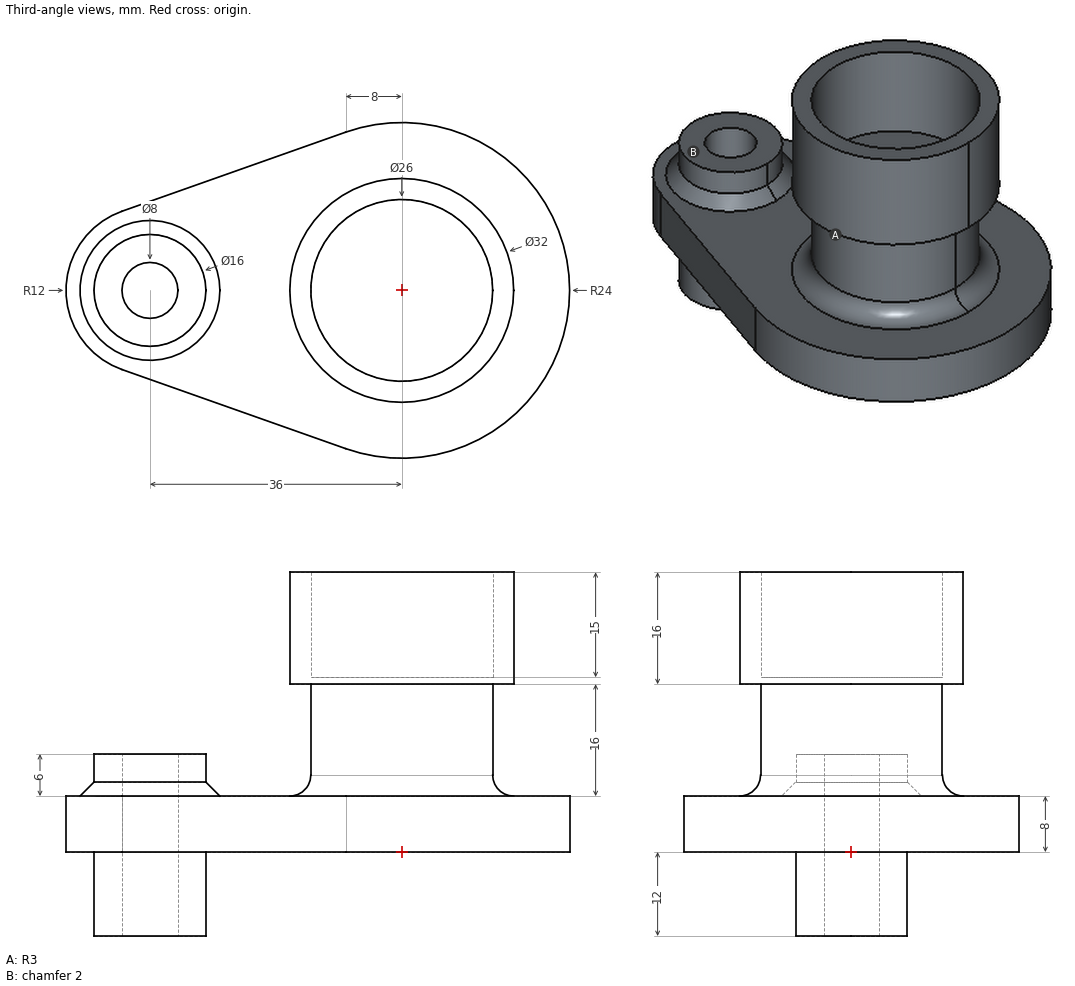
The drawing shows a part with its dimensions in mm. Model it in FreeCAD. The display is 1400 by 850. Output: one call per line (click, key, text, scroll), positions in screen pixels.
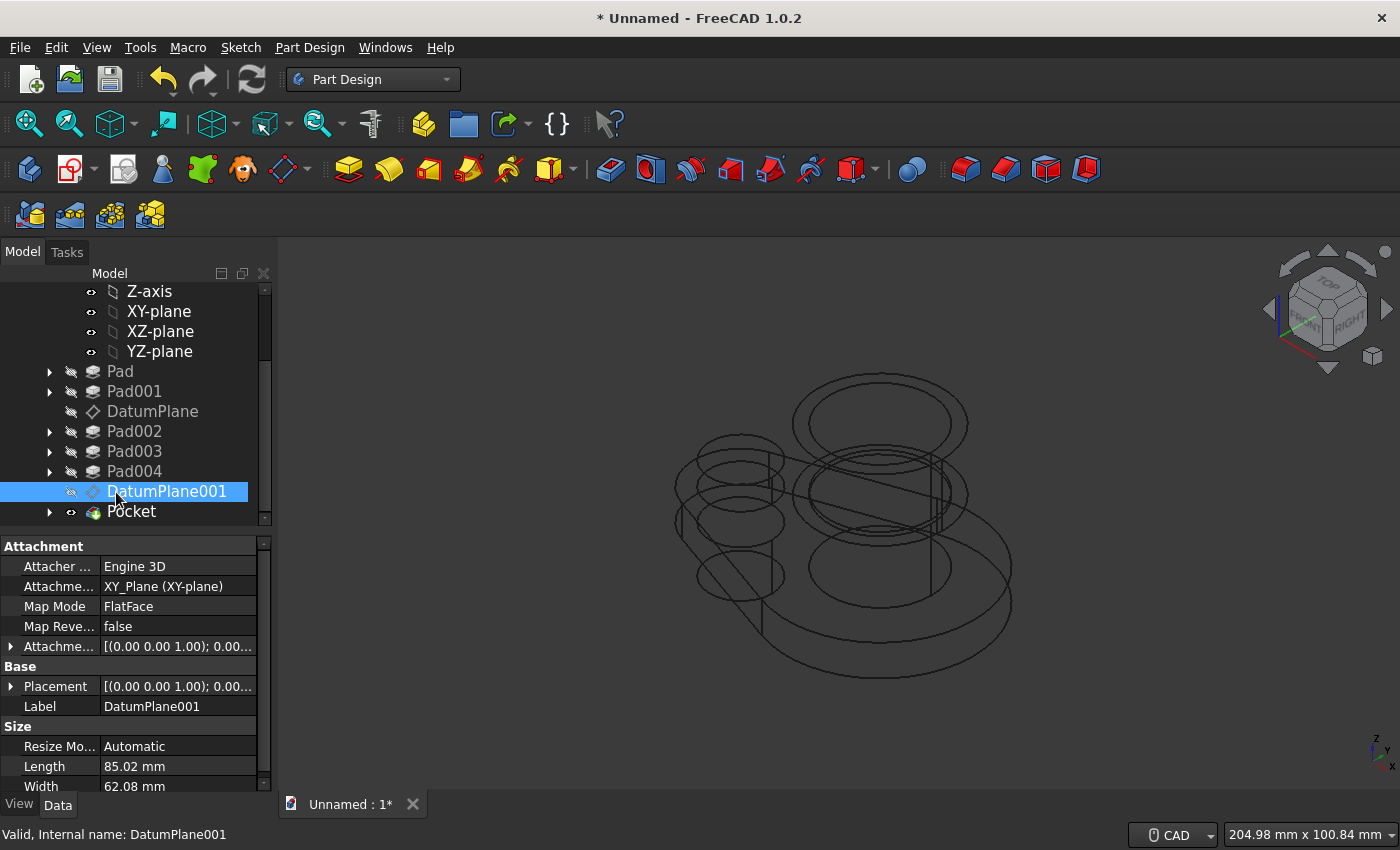
click(810, 560)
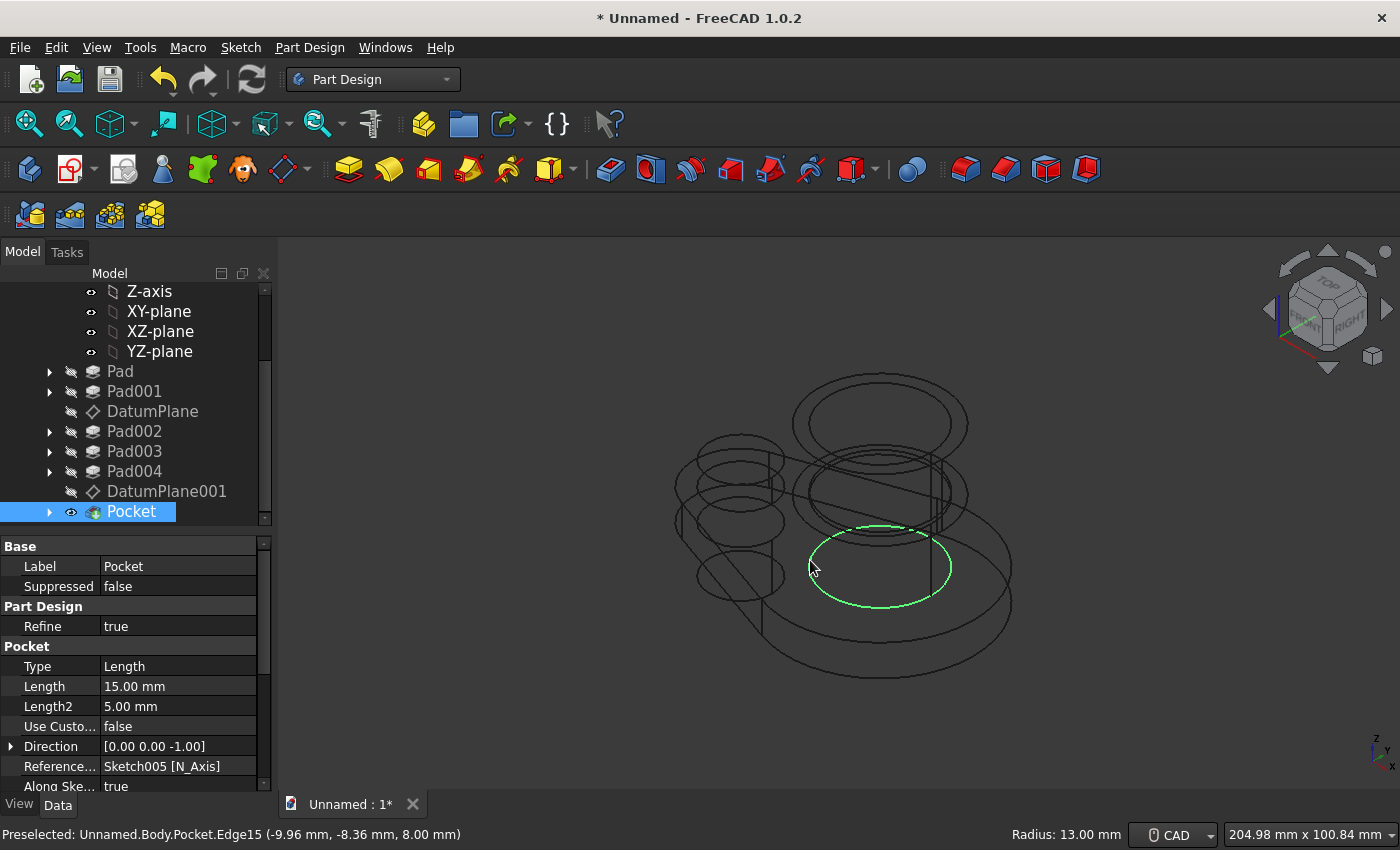
key(v)
key(1)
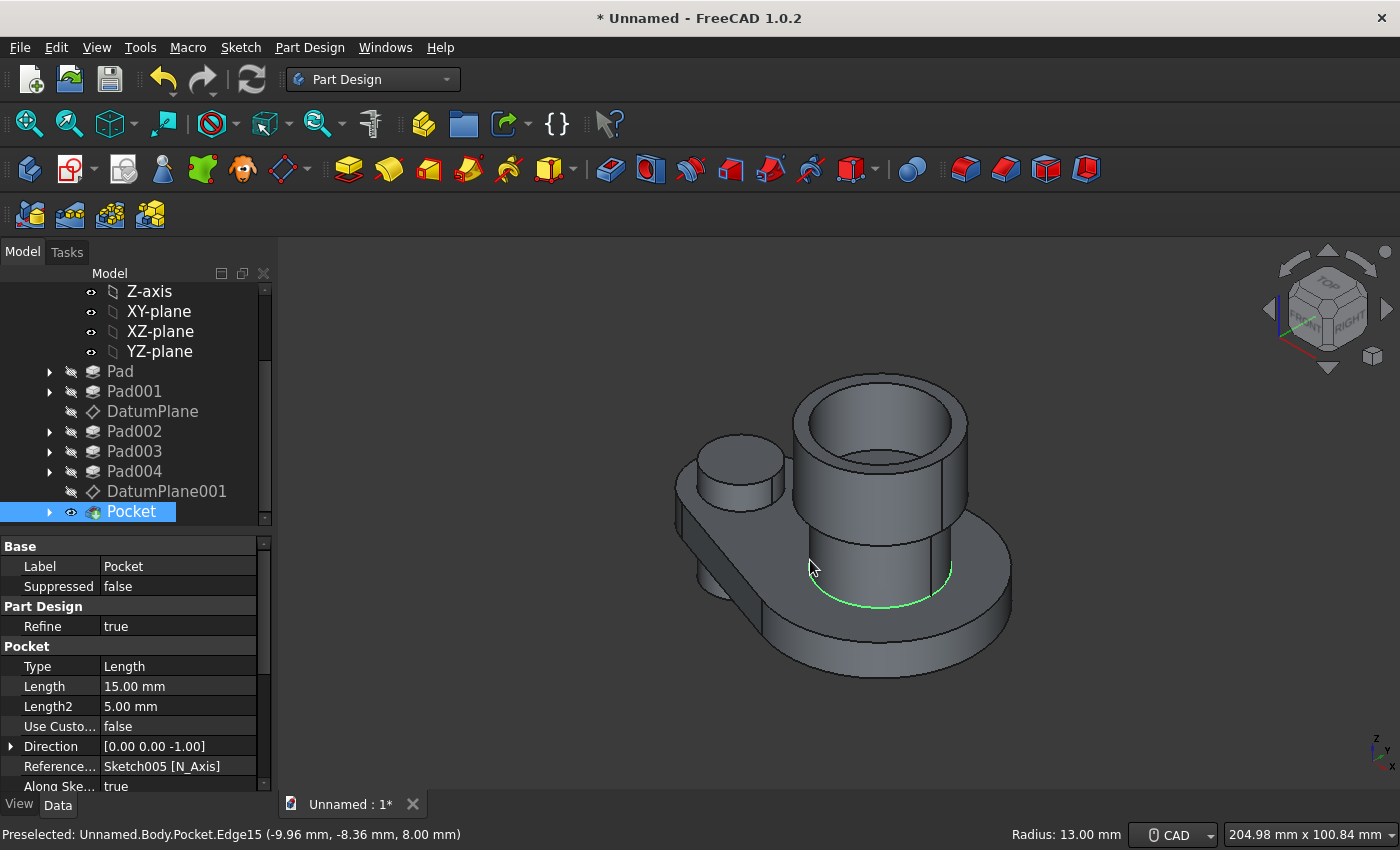
click(966, 170)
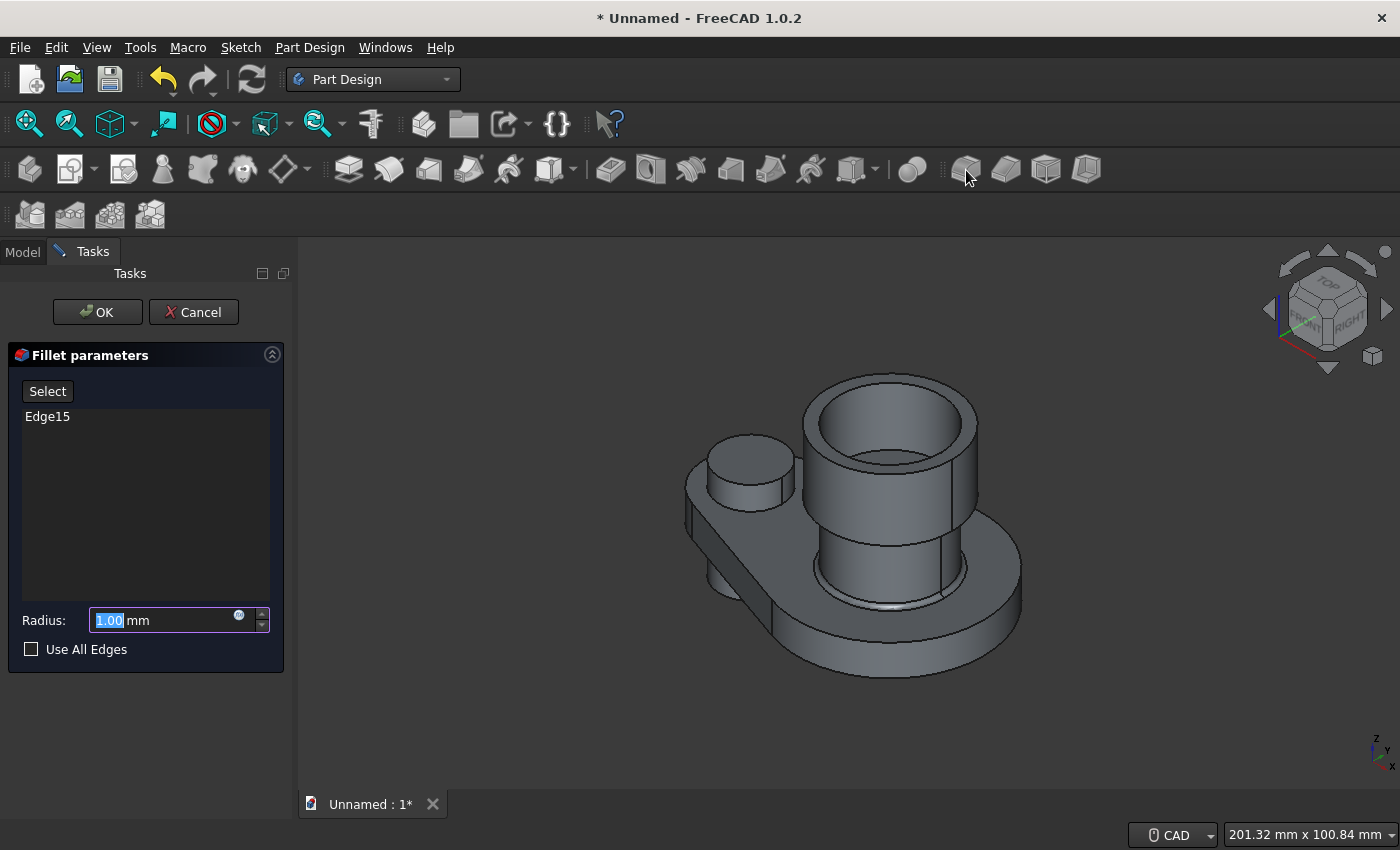
text(3)
key(Tab)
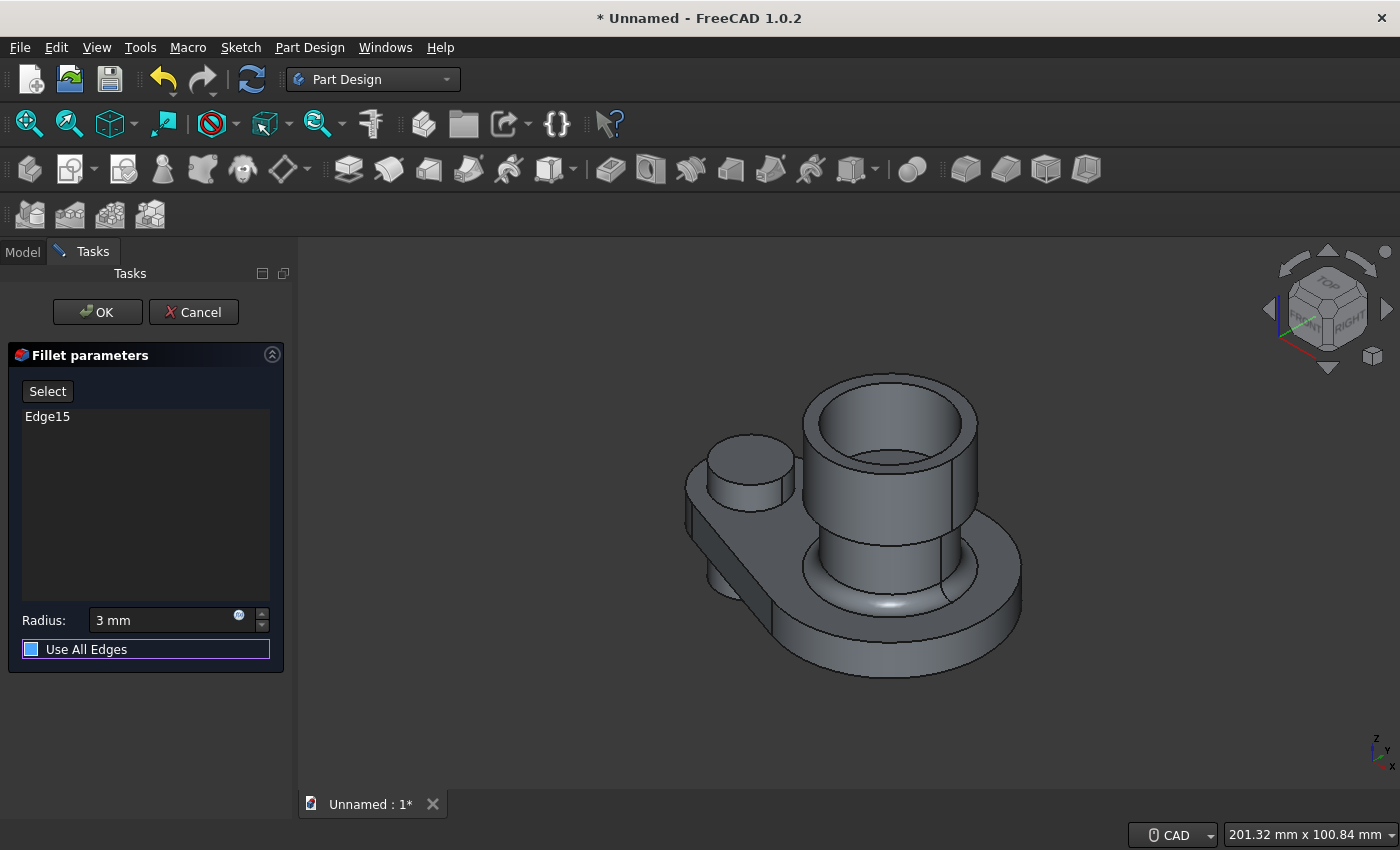
click(98, 312)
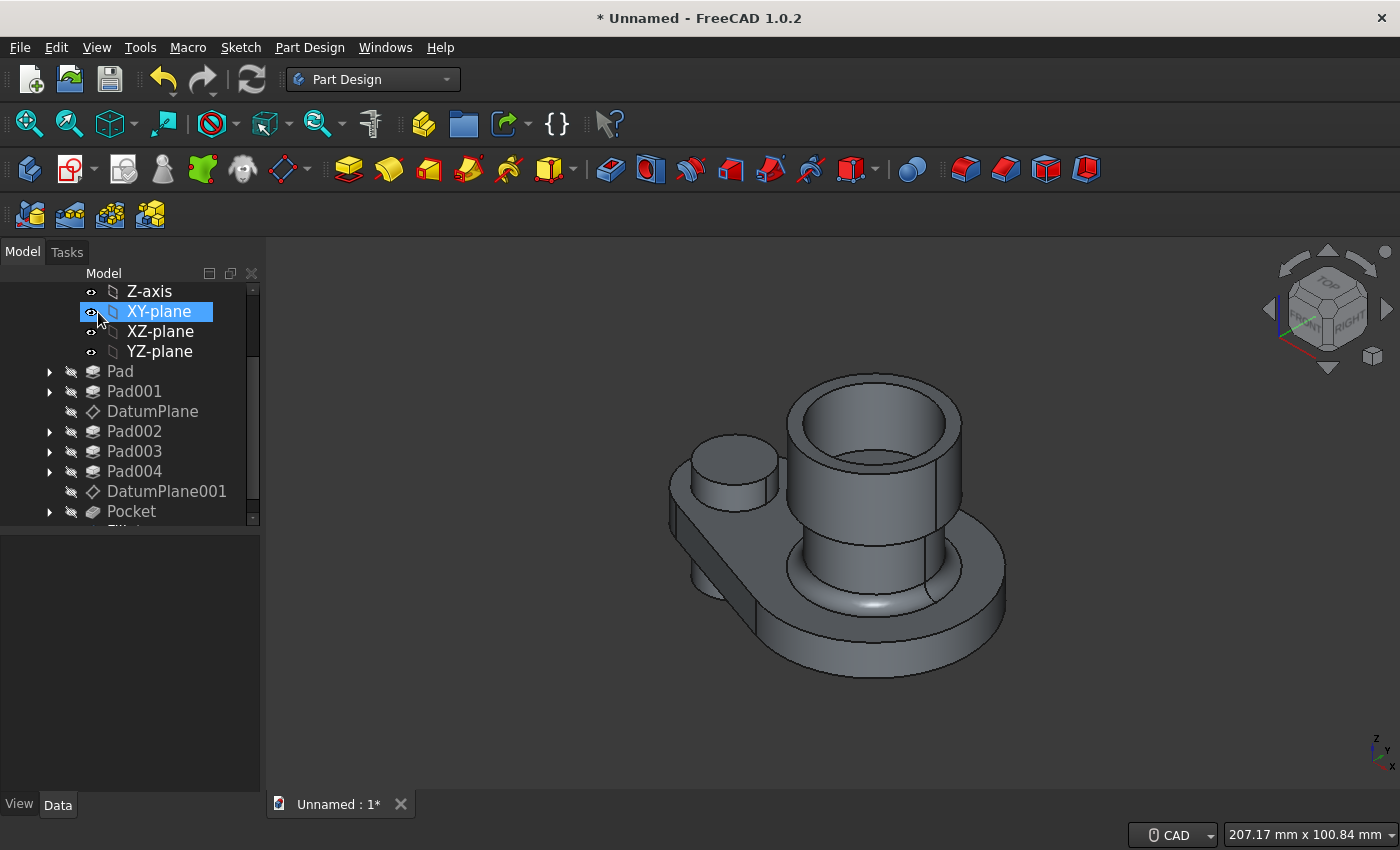
key(2)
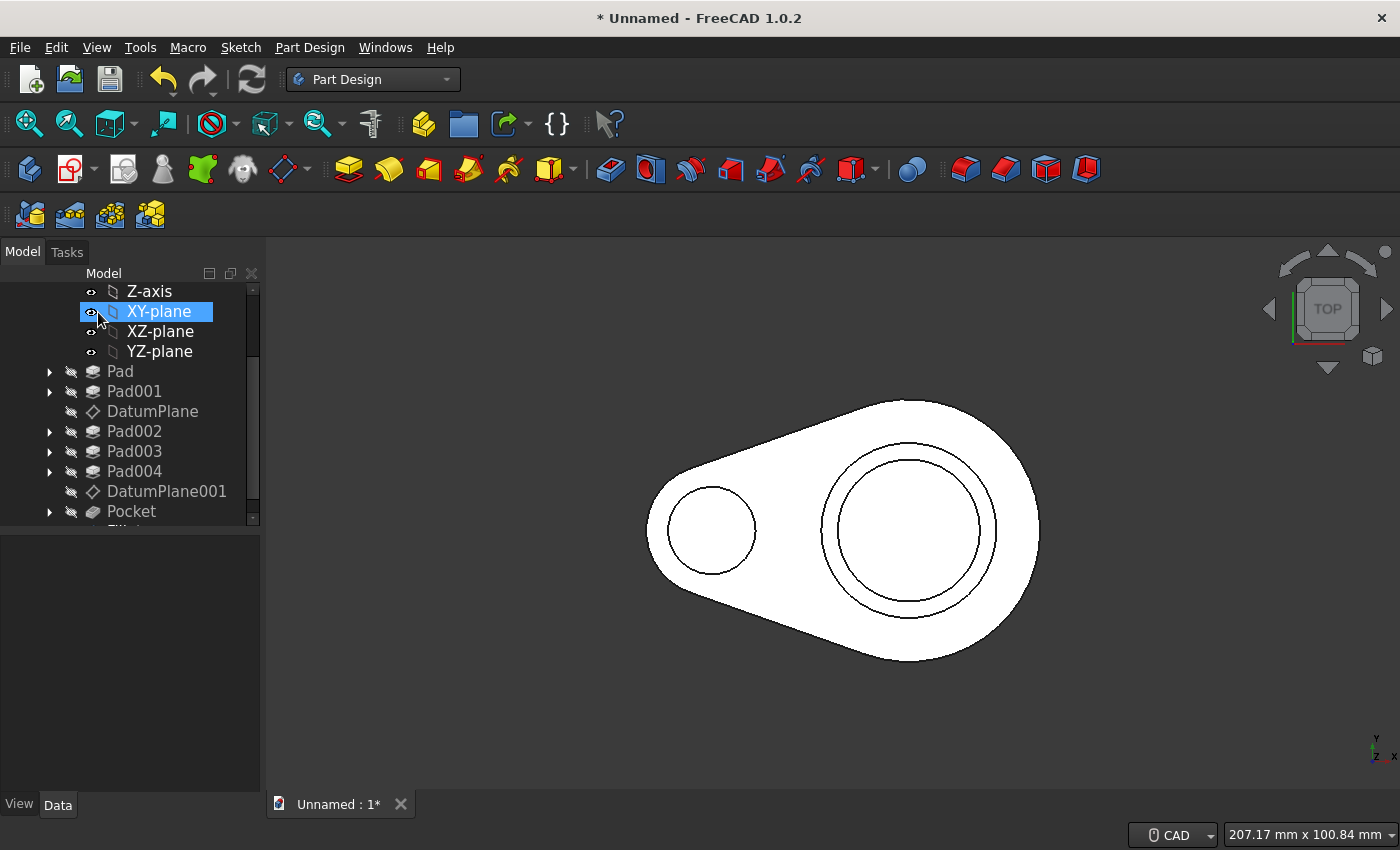
key(0)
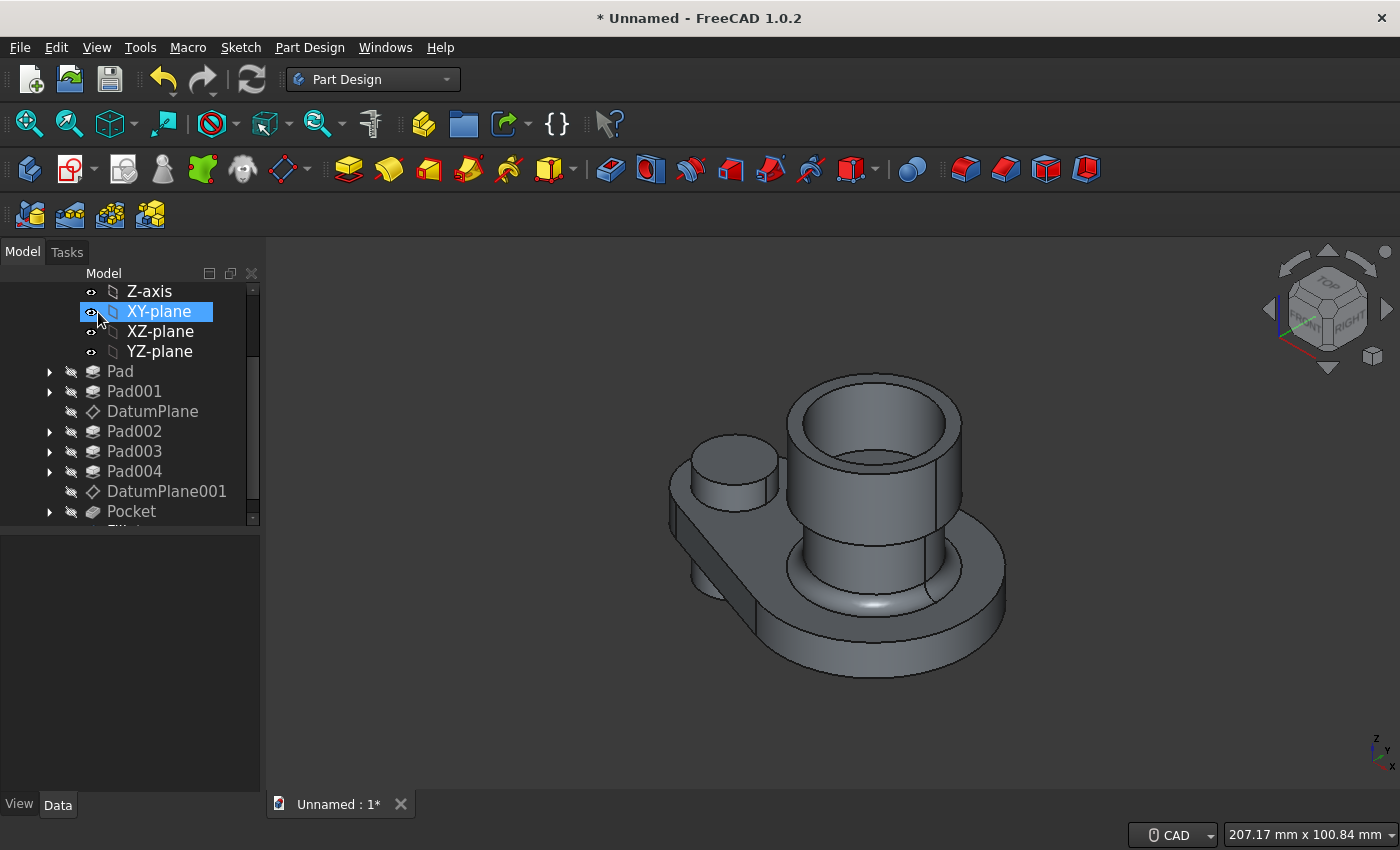
key(1)